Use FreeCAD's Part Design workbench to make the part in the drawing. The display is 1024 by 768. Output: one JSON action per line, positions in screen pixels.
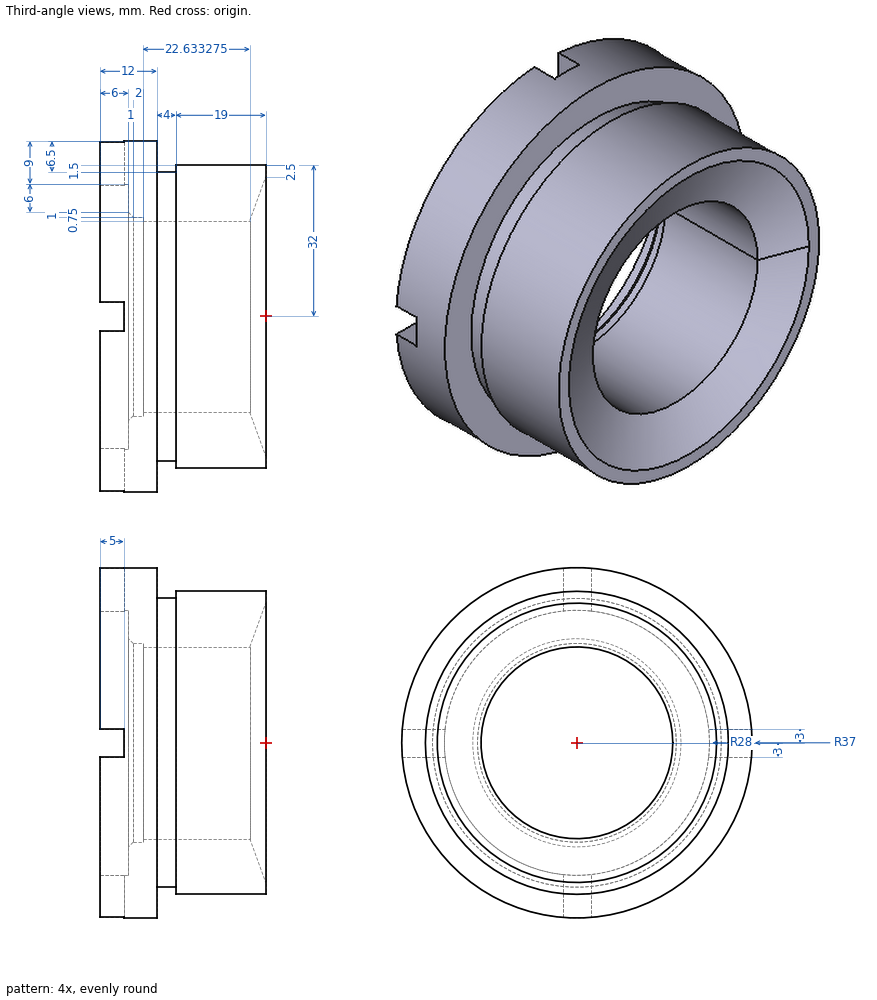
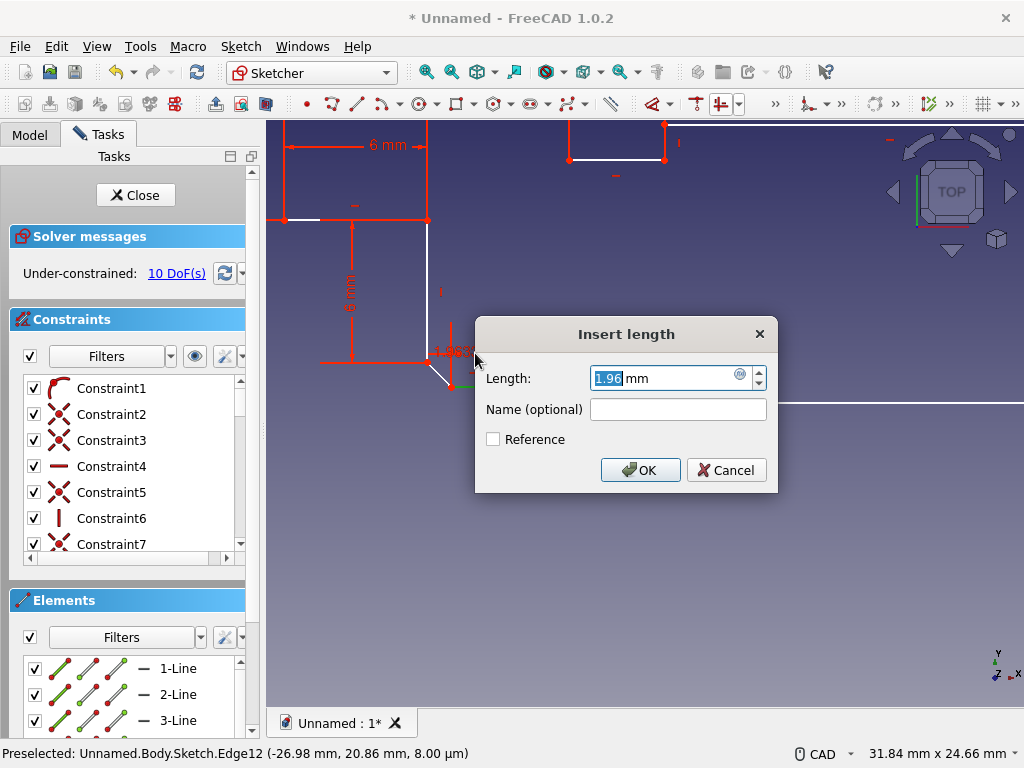
{"action": "type", "text": "2"}
{"action": "key", "text": "Return"}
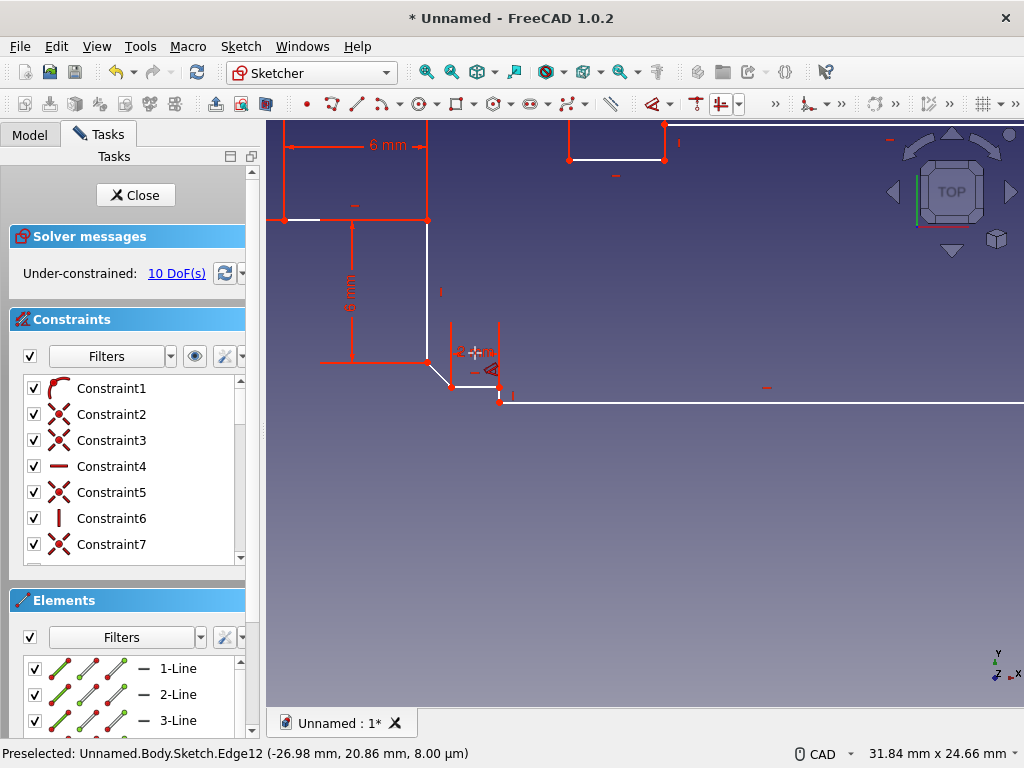
{"action": "scroll", "coordinate": [475, 389], "scroll_direction": "down", "scroll_amount": 4}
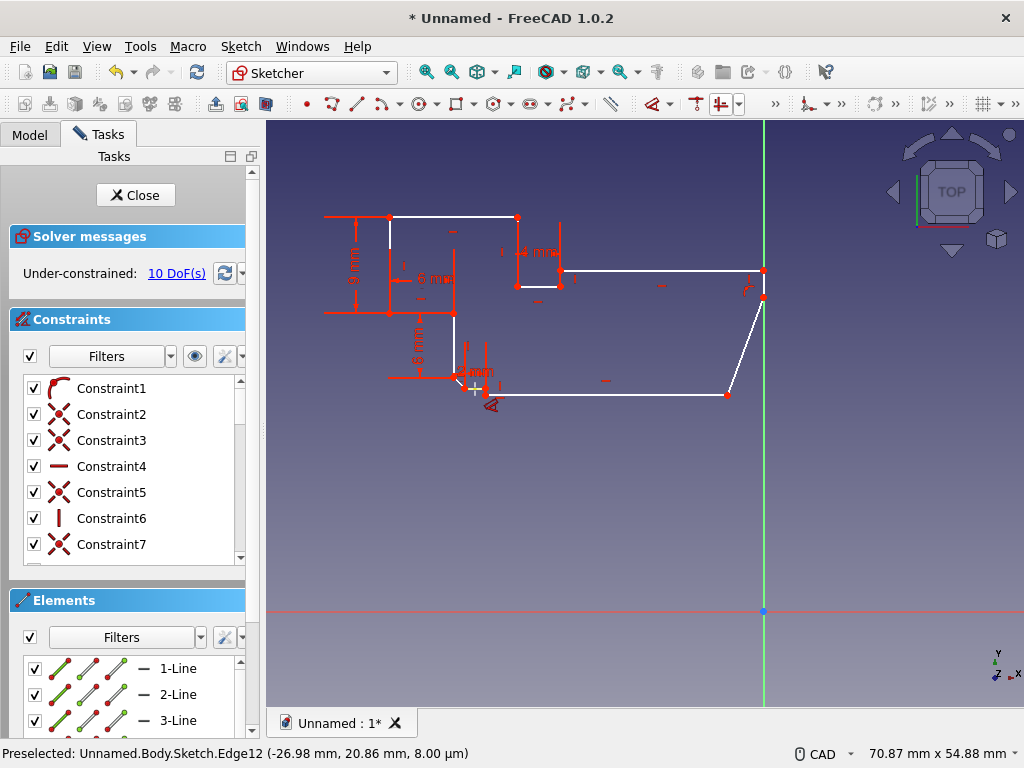
{"action": "left_click", "coordinate": [703, 271]}
{"action": "left_click", "coordinate": [662, 237]}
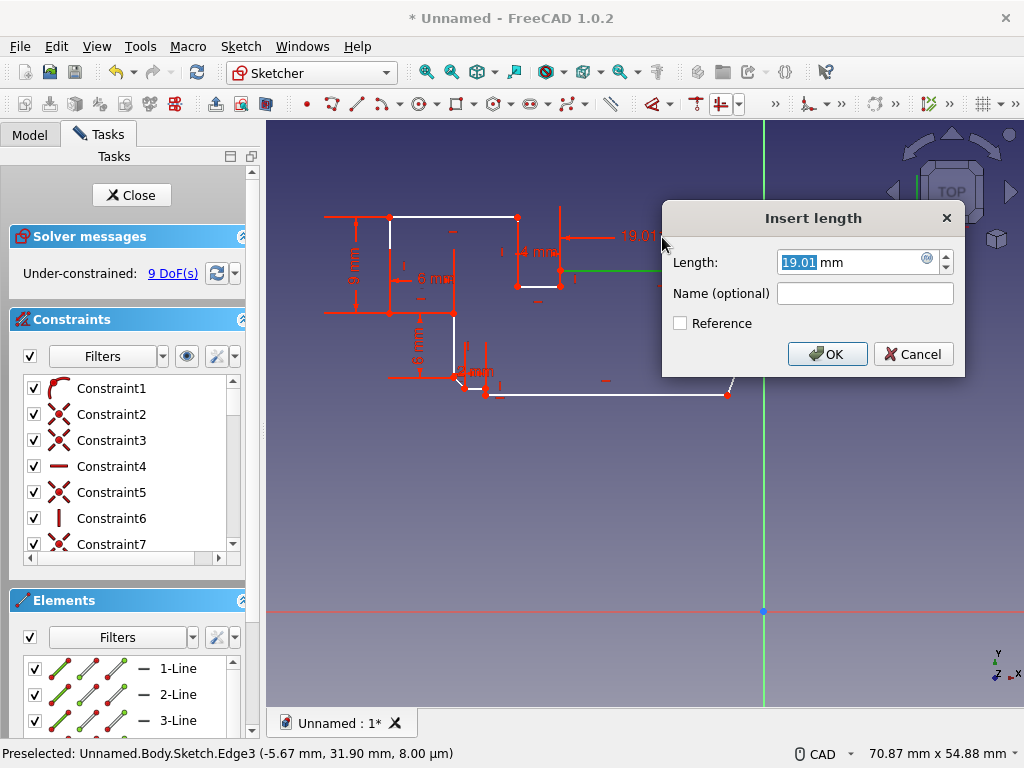
{"action": "type", "text": "19"}
{"action": "key", "text": "Return"}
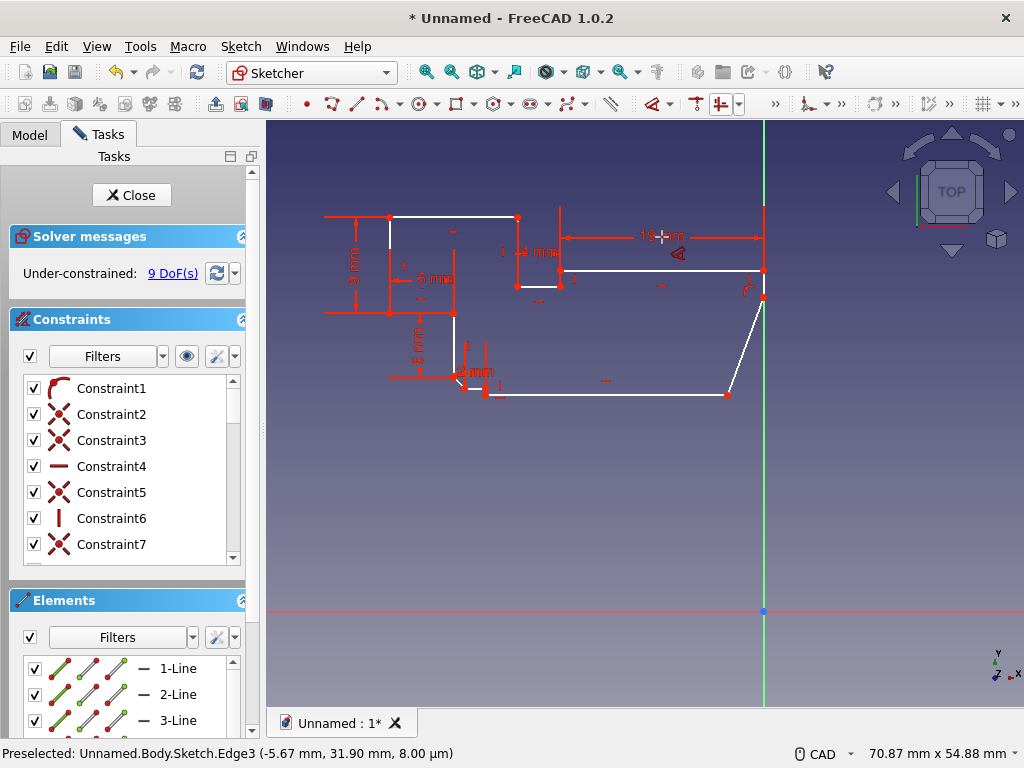
{"action": "left_click", "coordinate": [479, 217]}
{"action": "left_click", "coordinate": [454, 183]}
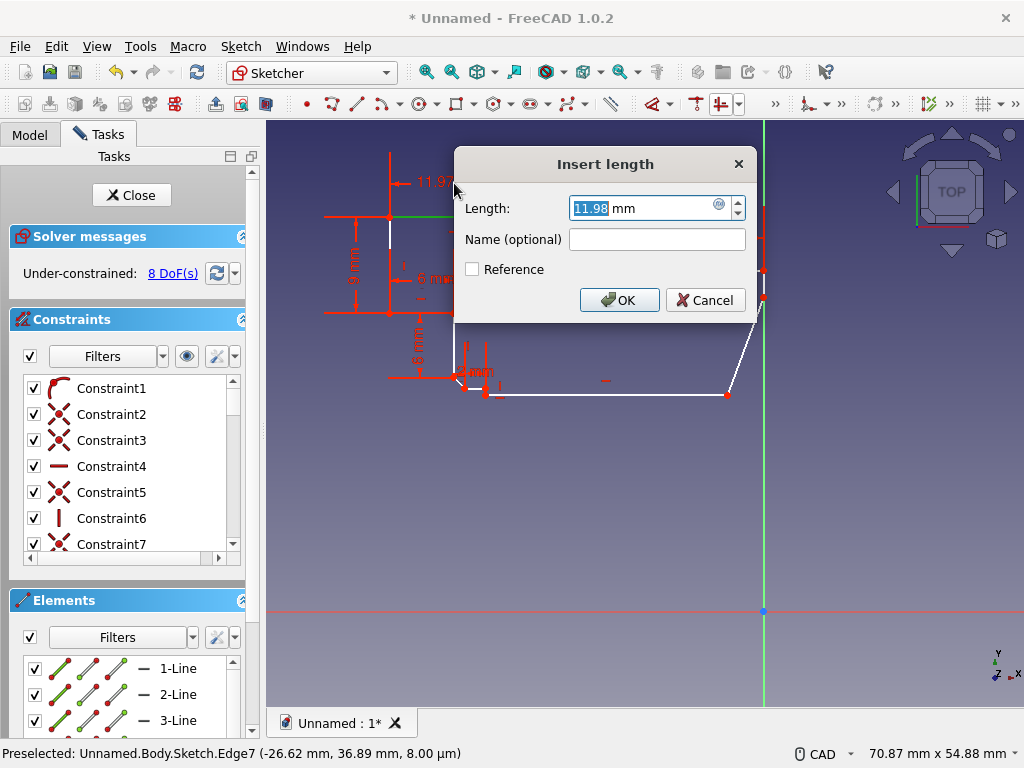
{"action": "type", "text": "12"}
{"action": "key", "text": "Return"}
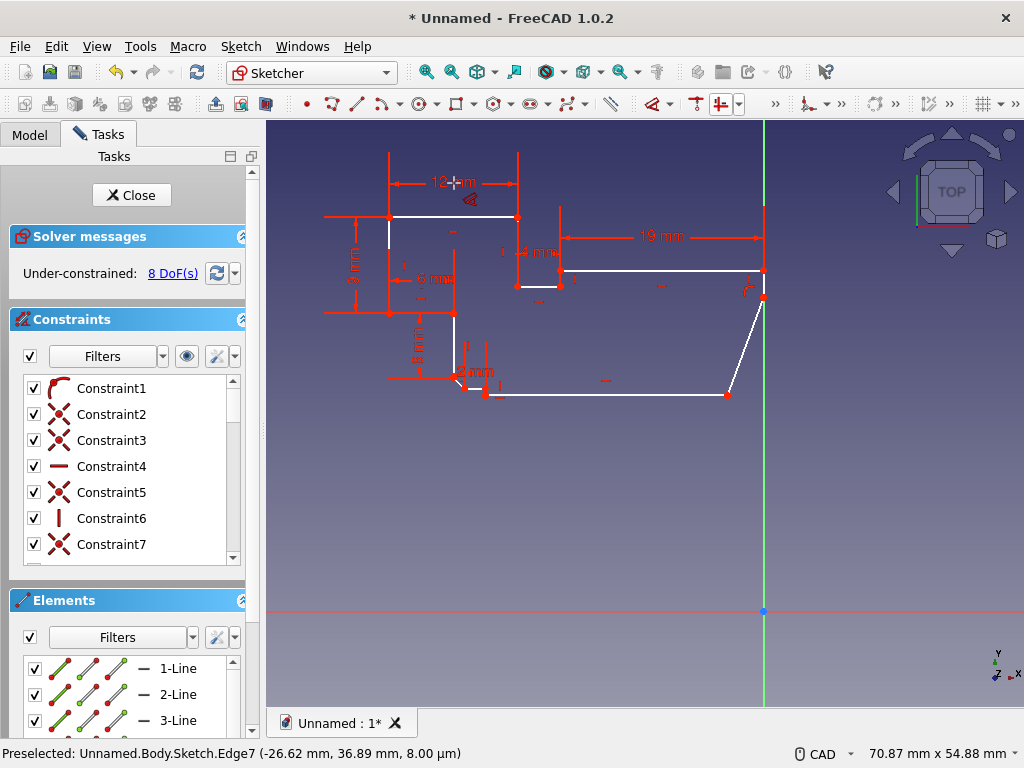
{"action": "scroll", "coordinate": [459, 383], "scroll_direction": "up", "scroll_amount": 7}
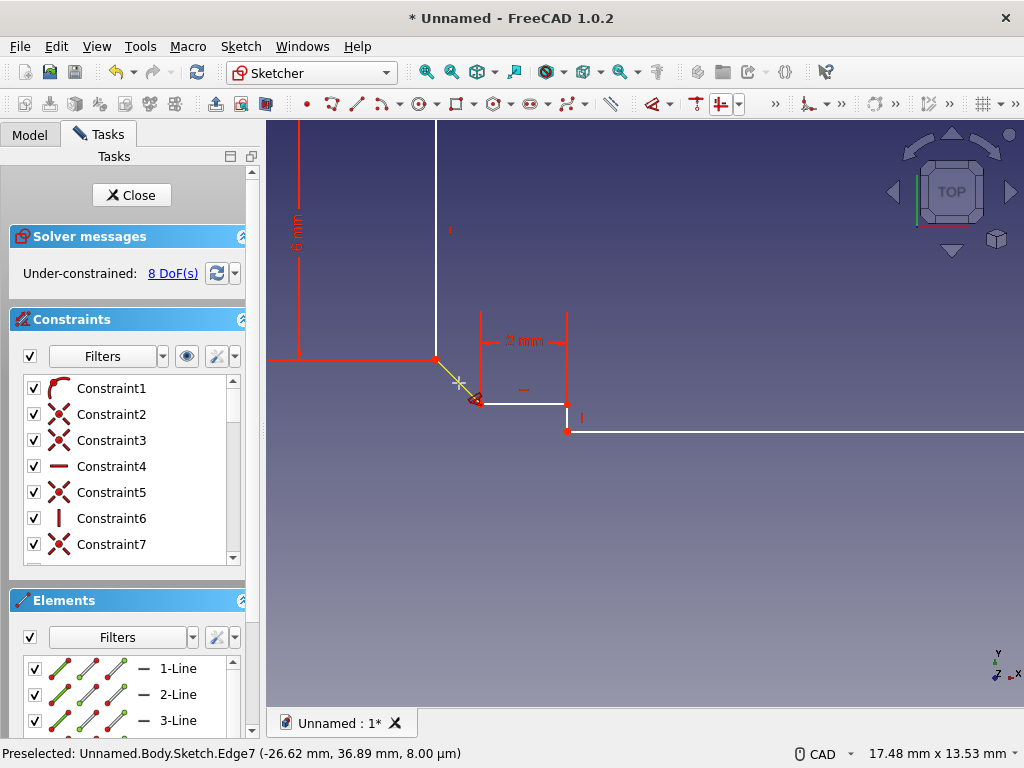
{"action": "left_click", "coordinate": [458, 382]}
{"action": "left_click", "coordinate": [458, 438]}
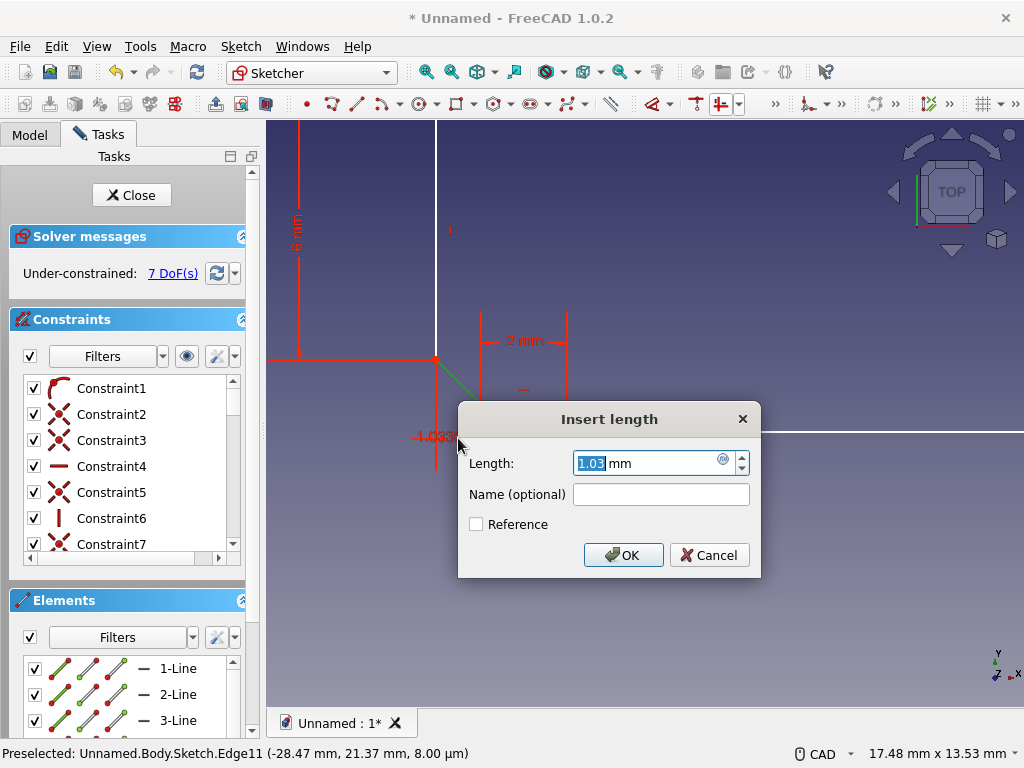
{"action": "type", "text": "1"}
{"action": "key", "text": "Return"}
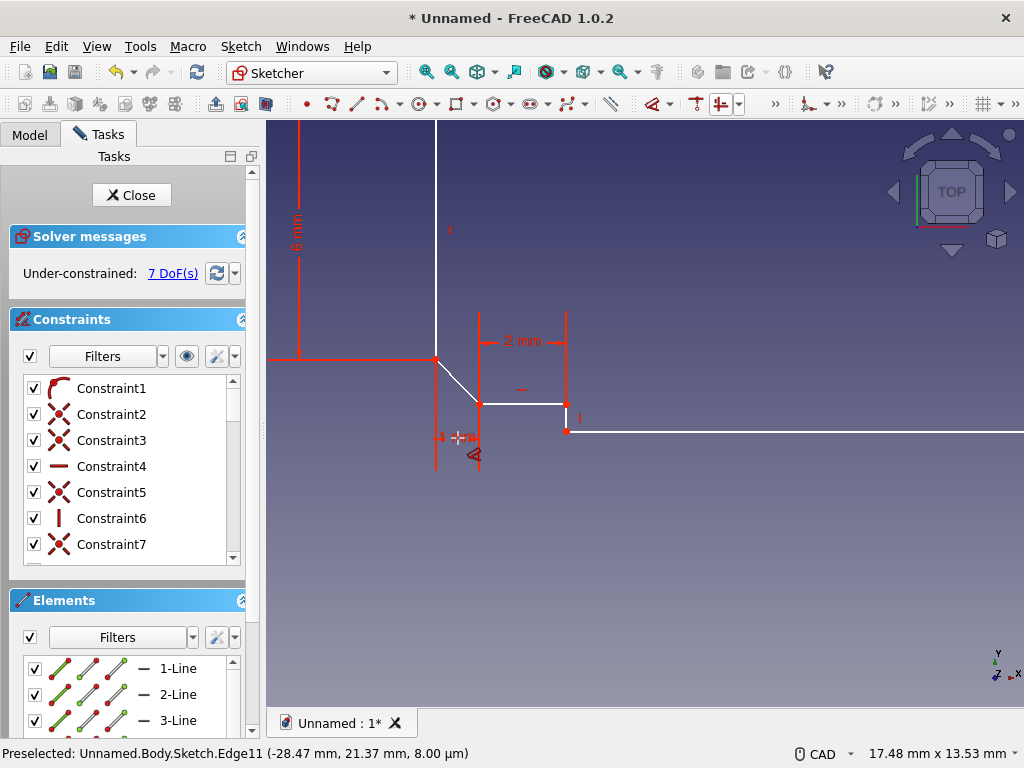
{"action": "left_click", "coordinate": [449, 373]}
{"action": "left_click", "coordinate": [402, 382]}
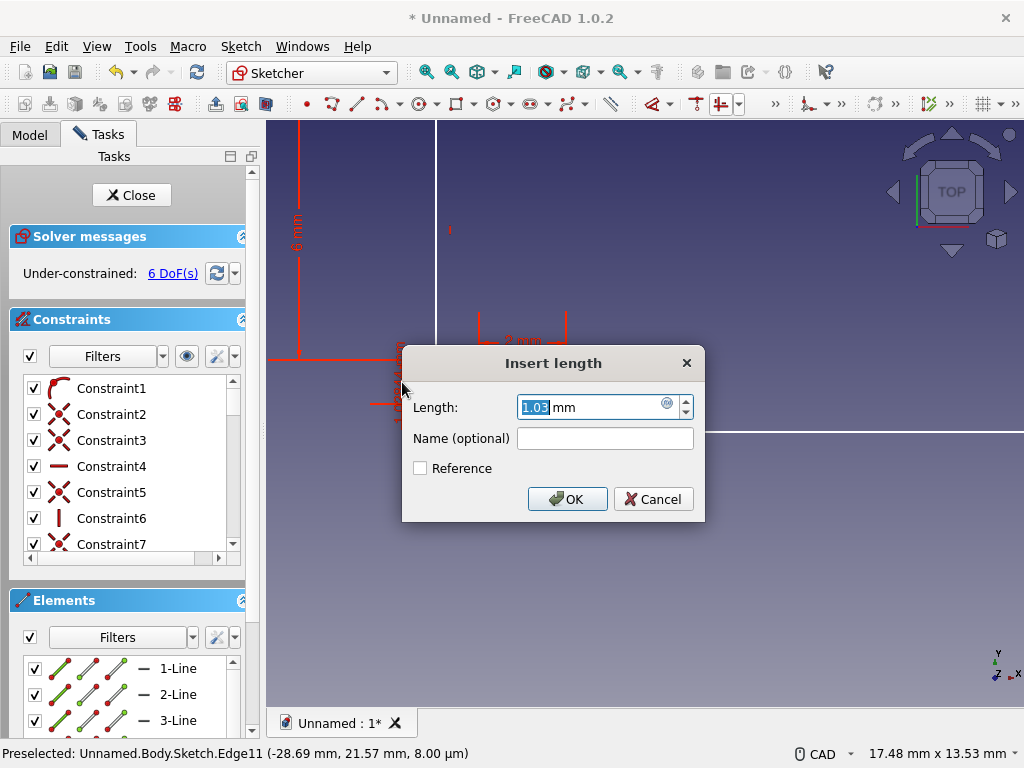
{"action": "type", "text": "1"}
{"action": "key", "text": "Return"}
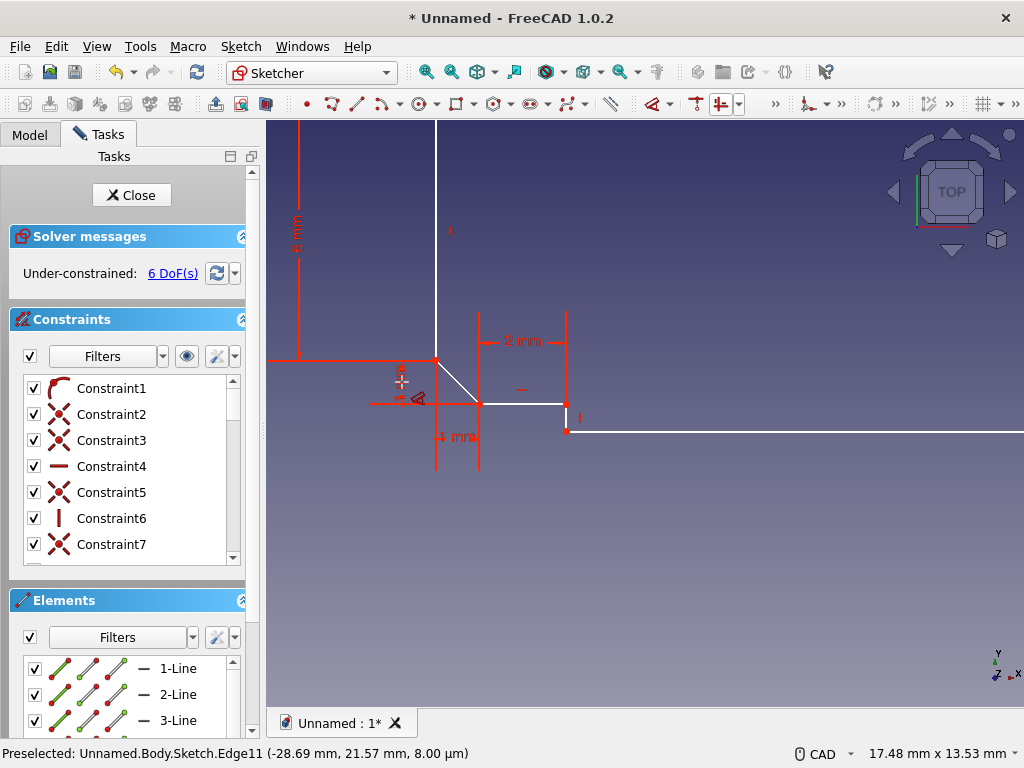
{"action": "scroll", "coordinate": [459, 383], "scroll_direction": "down", "scroll_amount": 7}